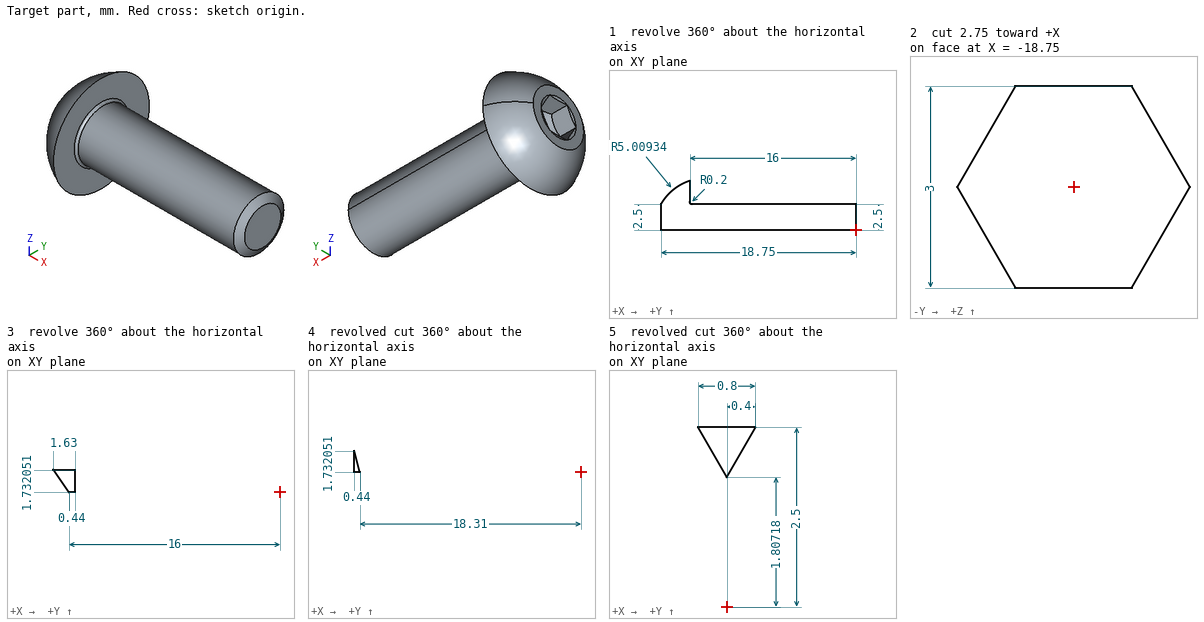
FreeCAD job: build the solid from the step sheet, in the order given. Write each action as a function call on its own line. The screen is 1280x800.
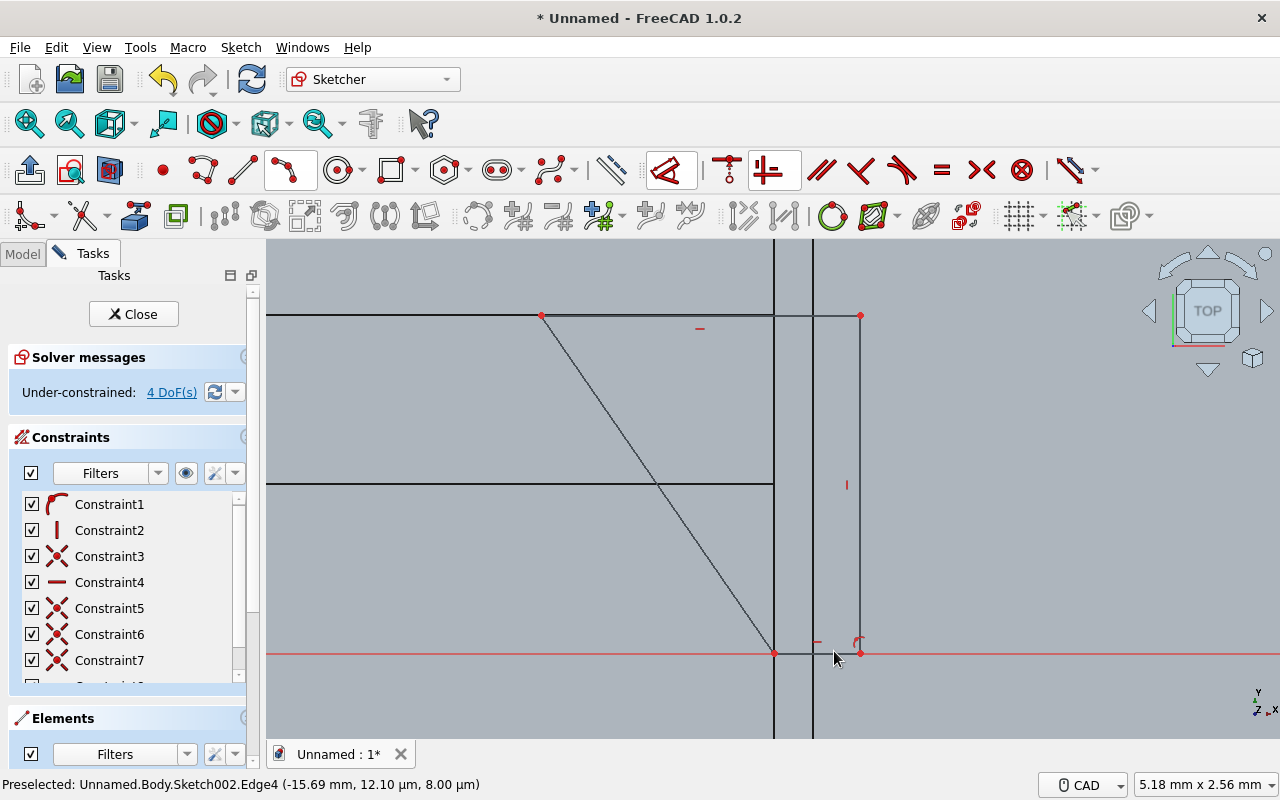
click(774, 654)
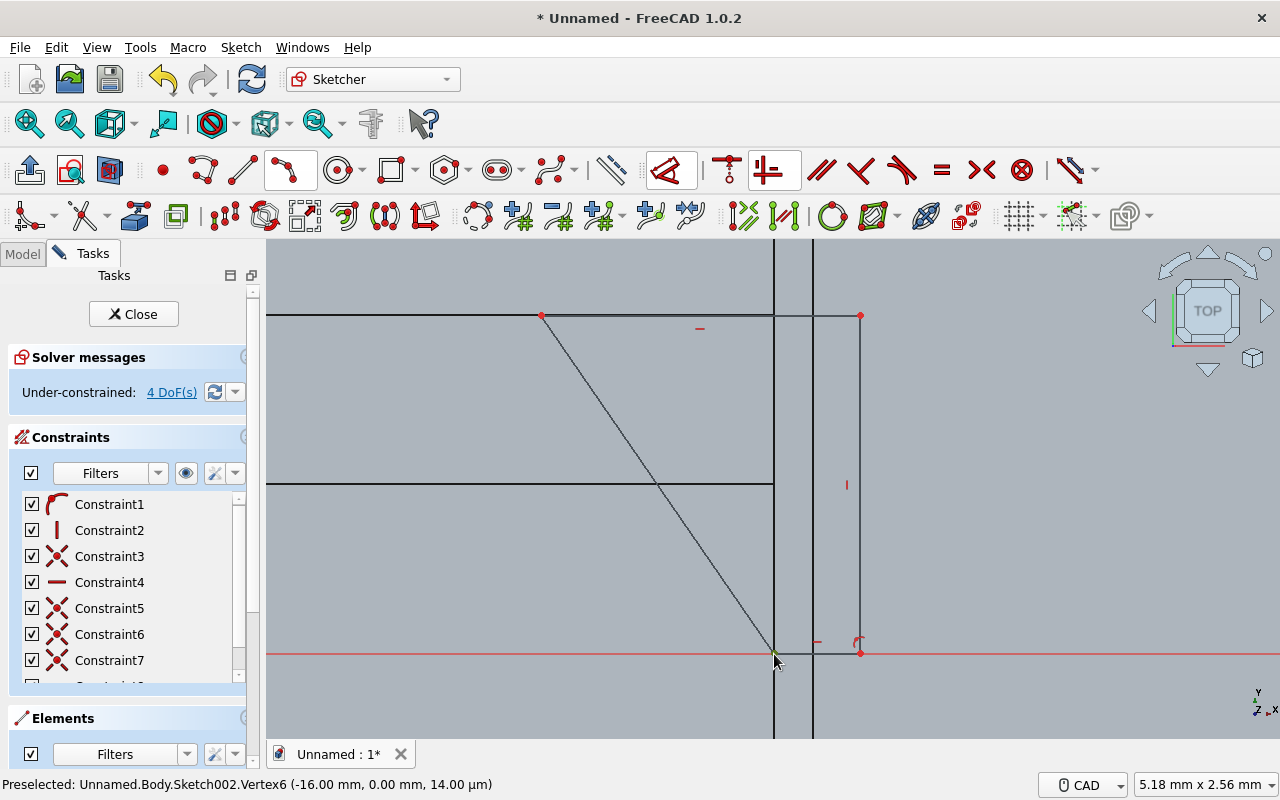
click(692, 170)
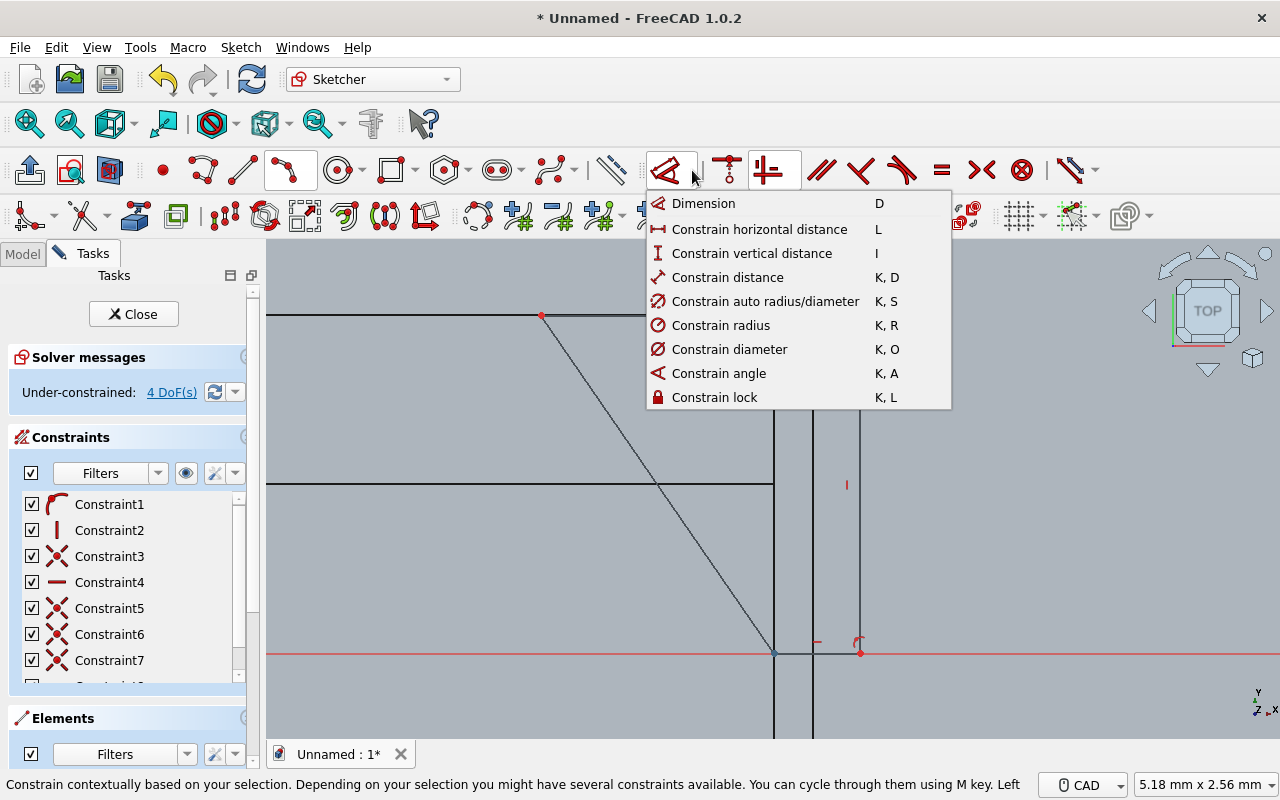
click(799, 229)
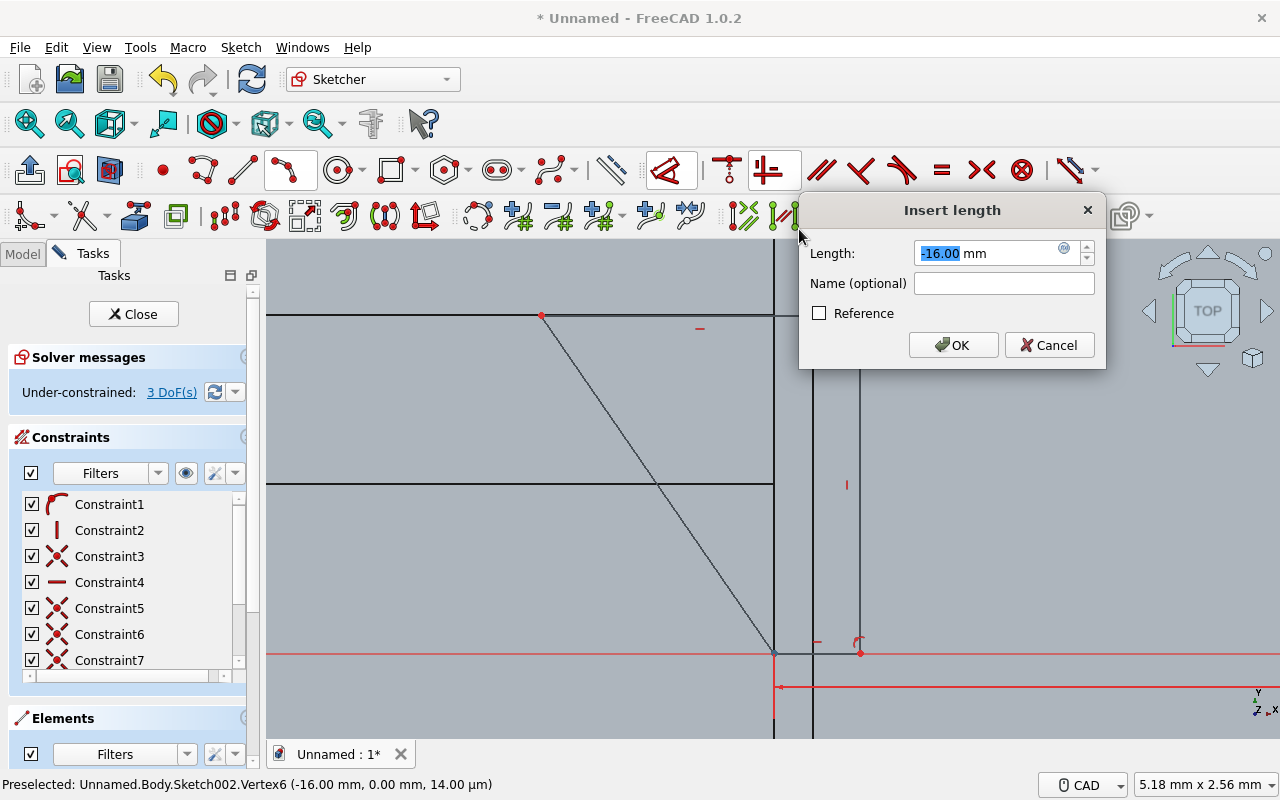
text(-16)
key(Return)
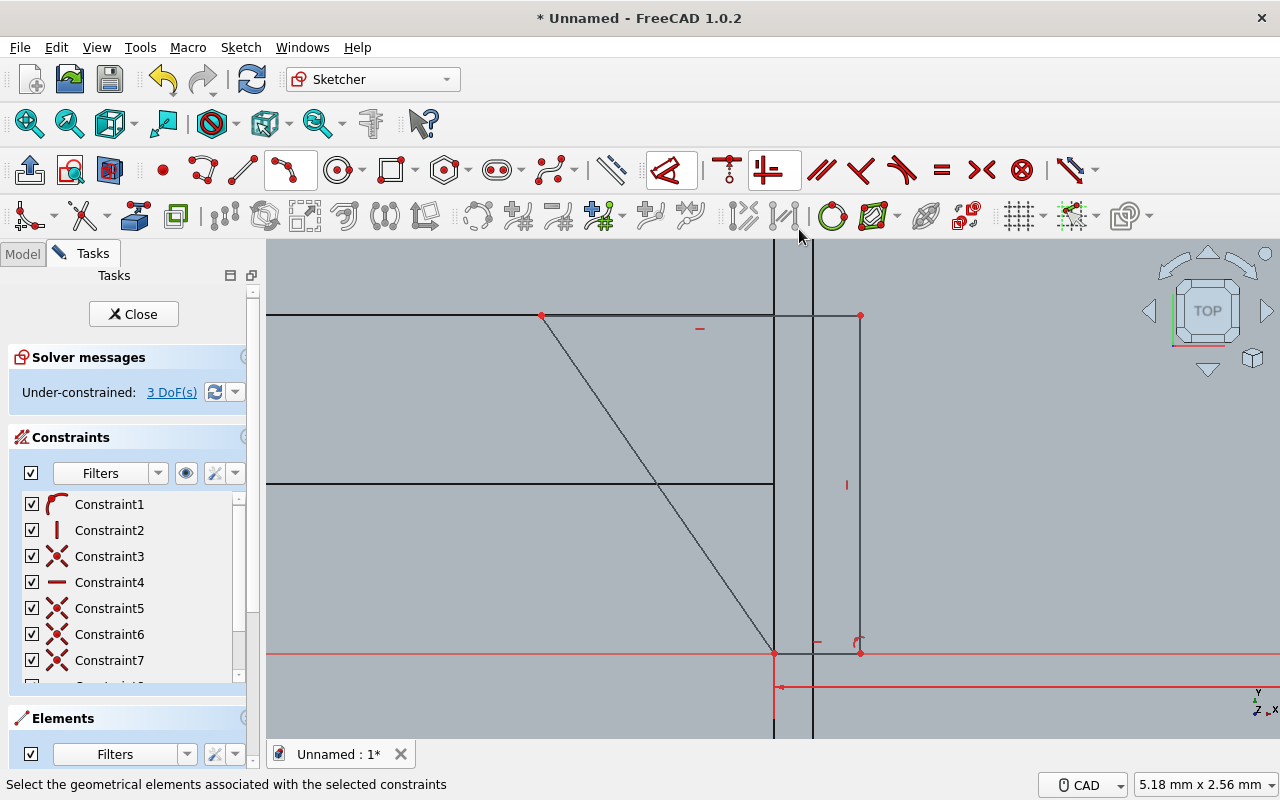
click(764, 316)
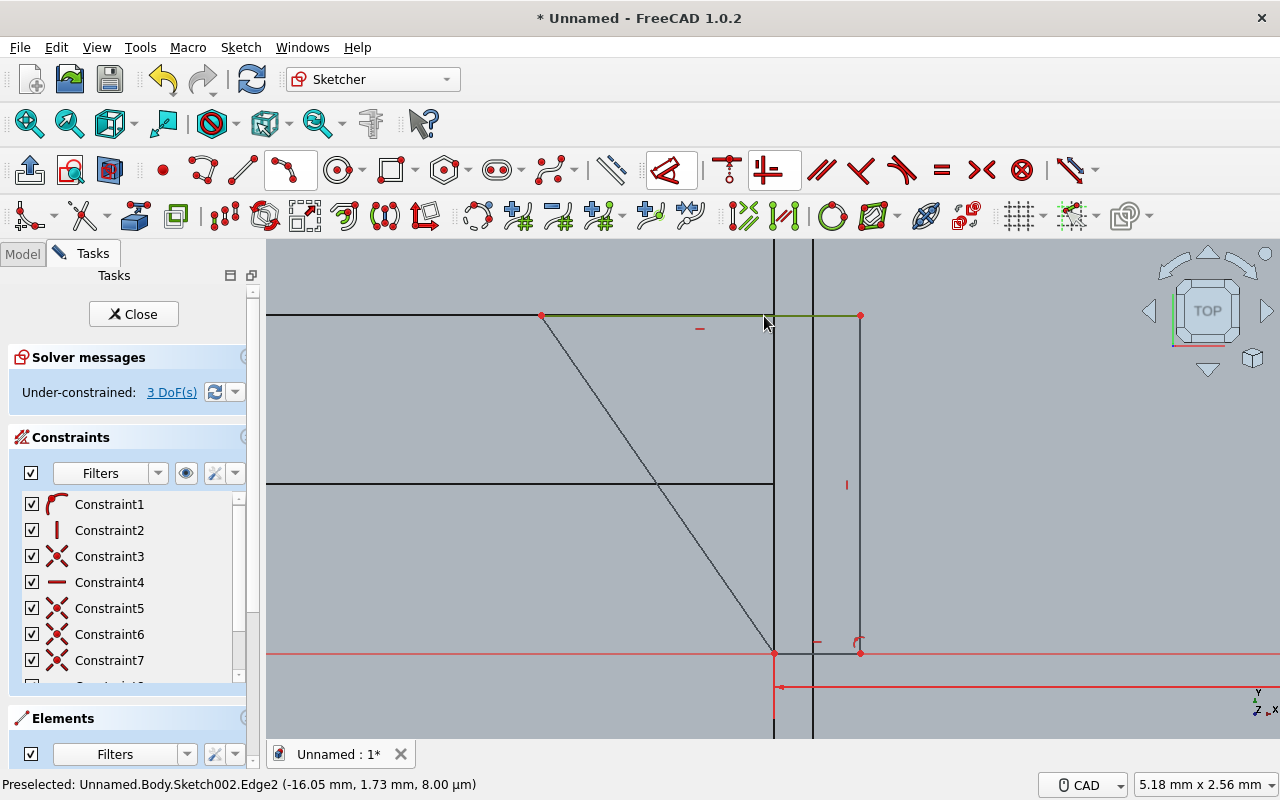
key(l)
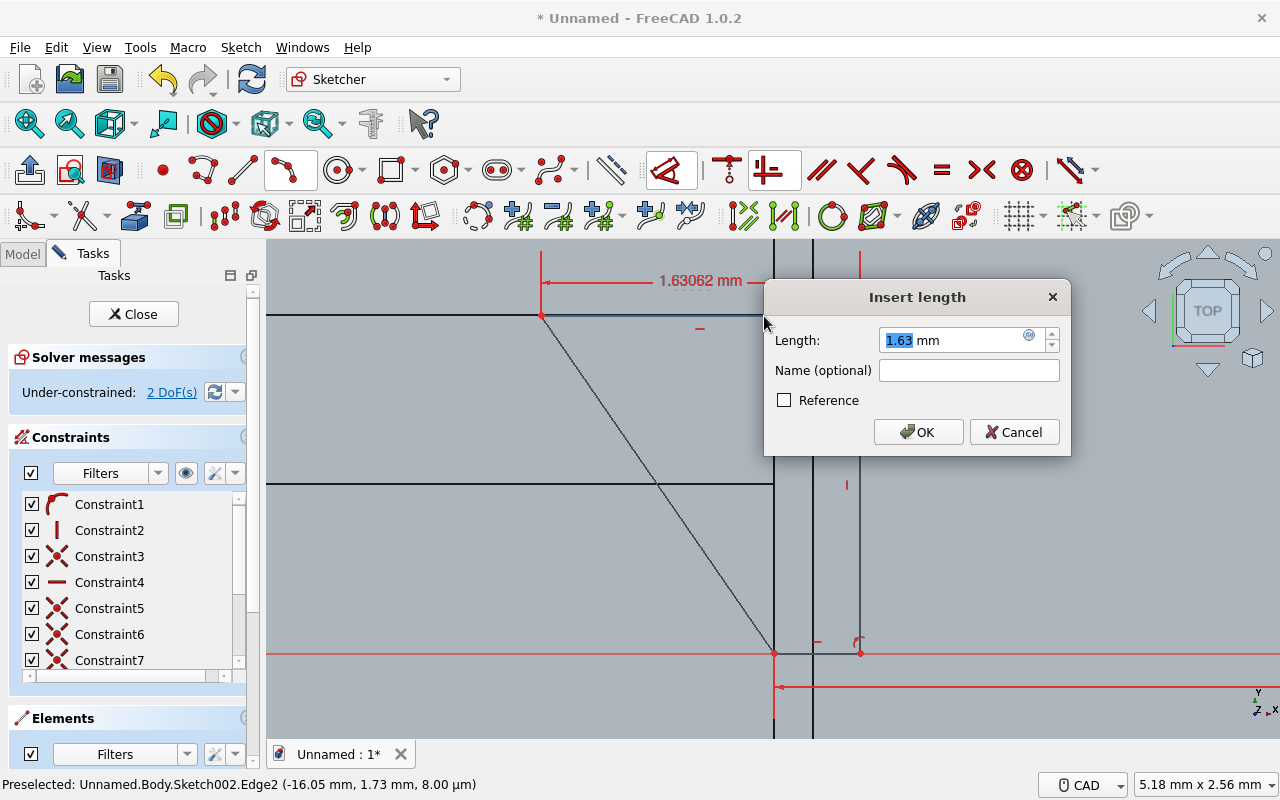
text(1.63)
key(Return)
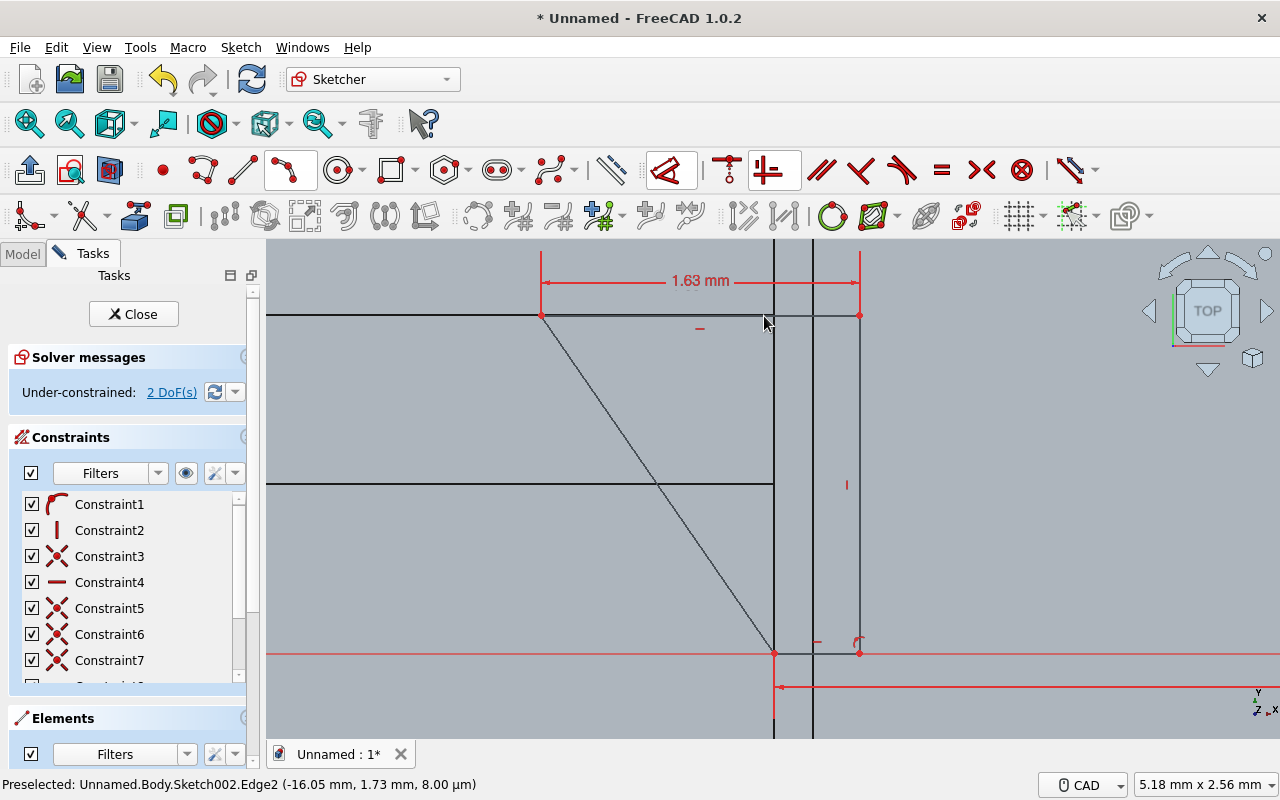
click(800, 654)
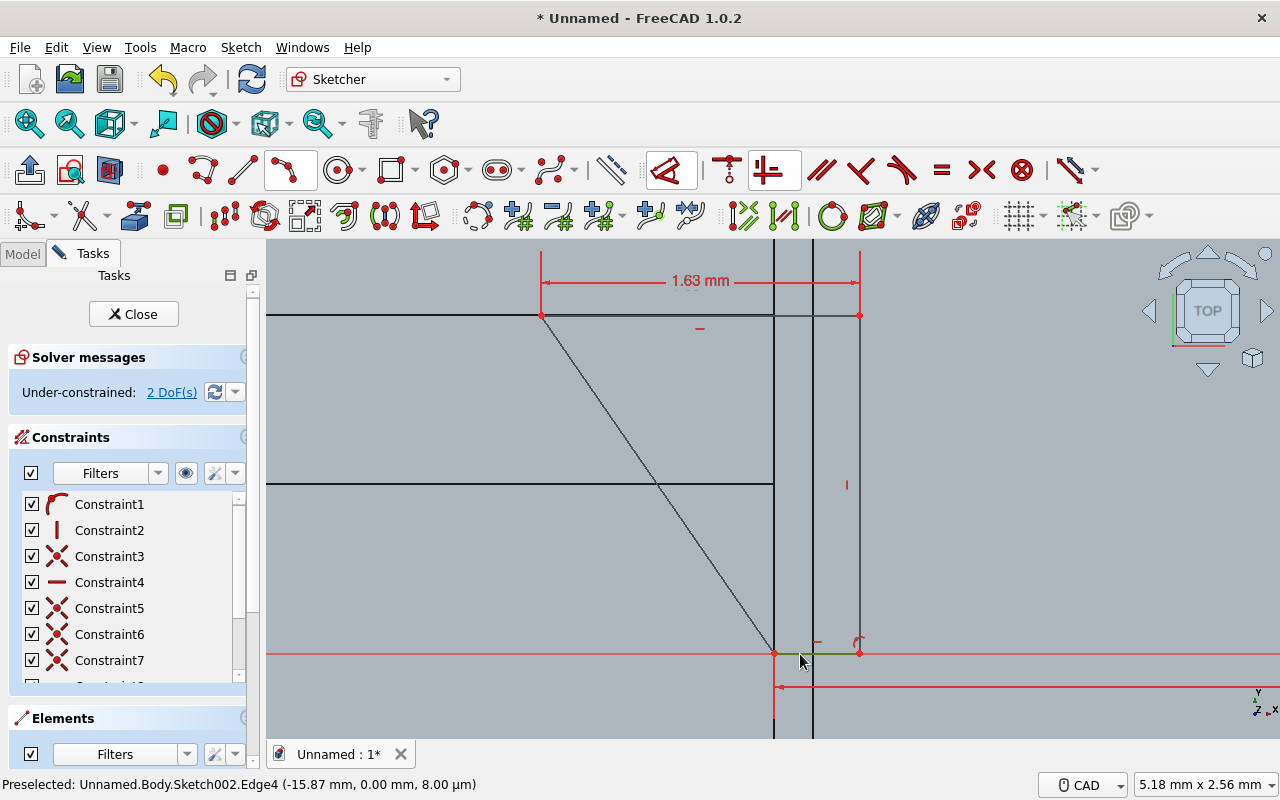
key(l)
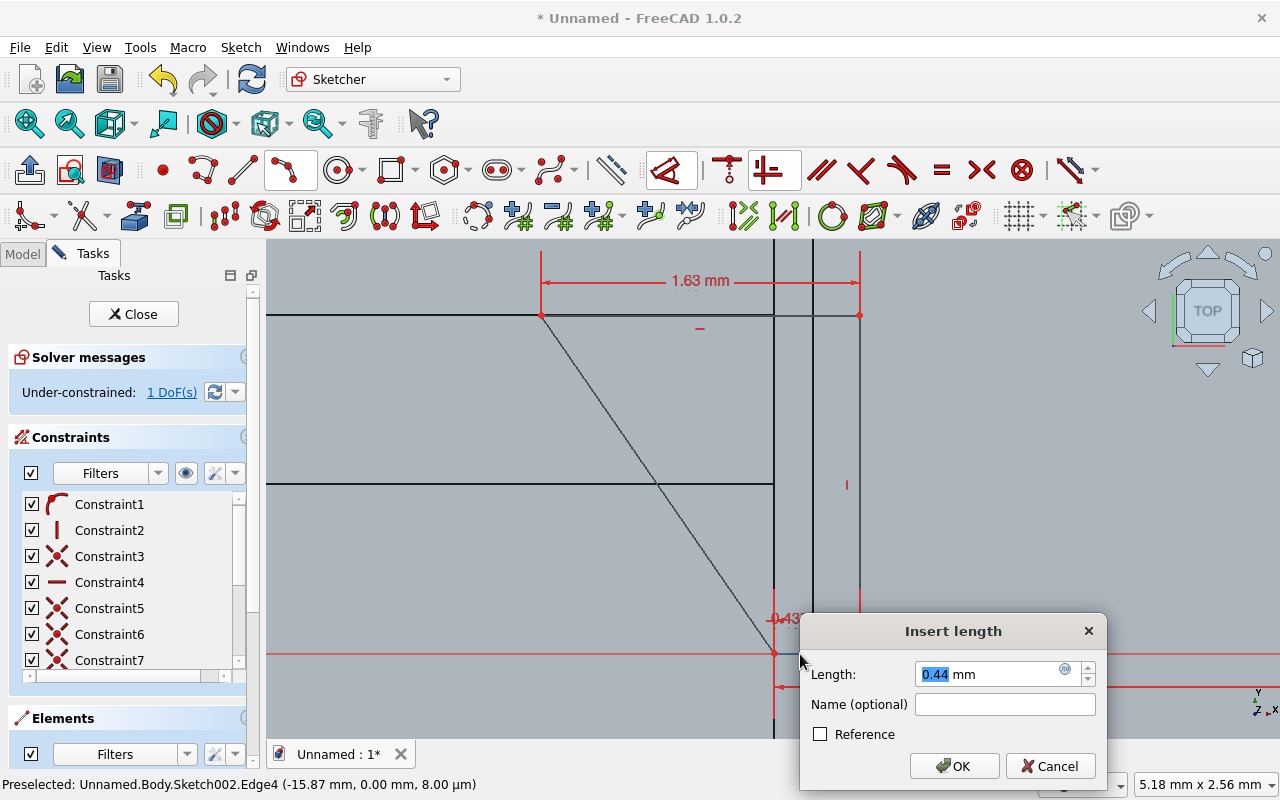
text(0.44)
key(Return)